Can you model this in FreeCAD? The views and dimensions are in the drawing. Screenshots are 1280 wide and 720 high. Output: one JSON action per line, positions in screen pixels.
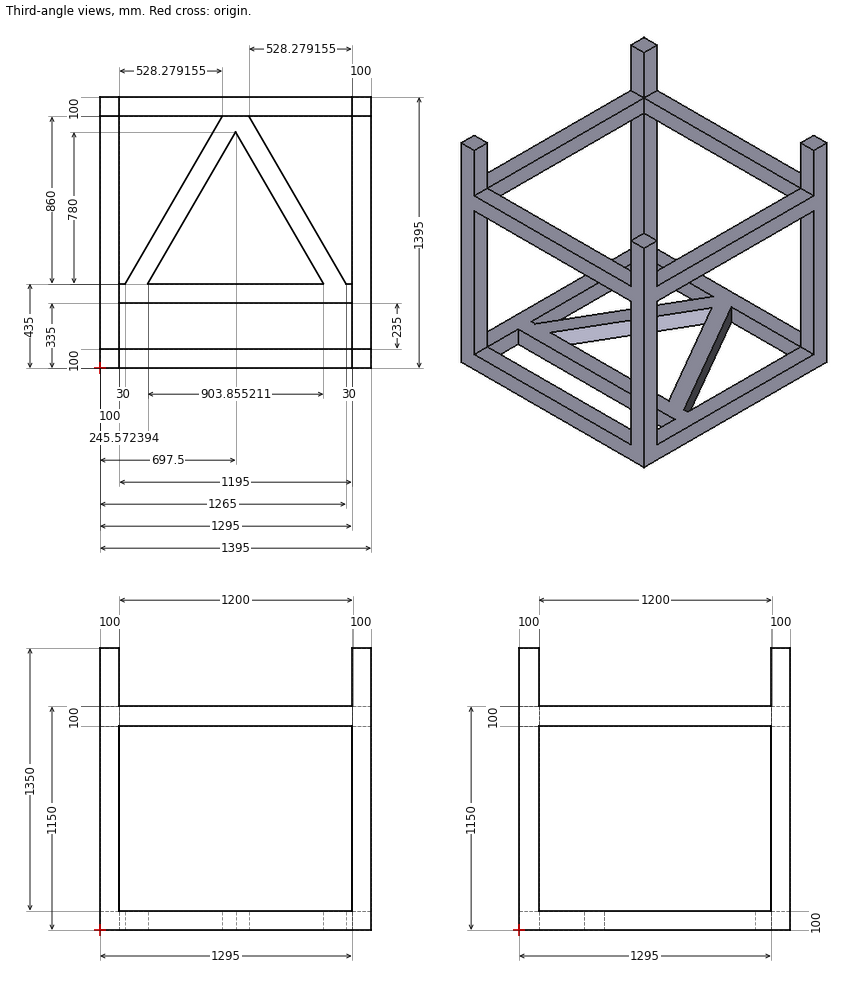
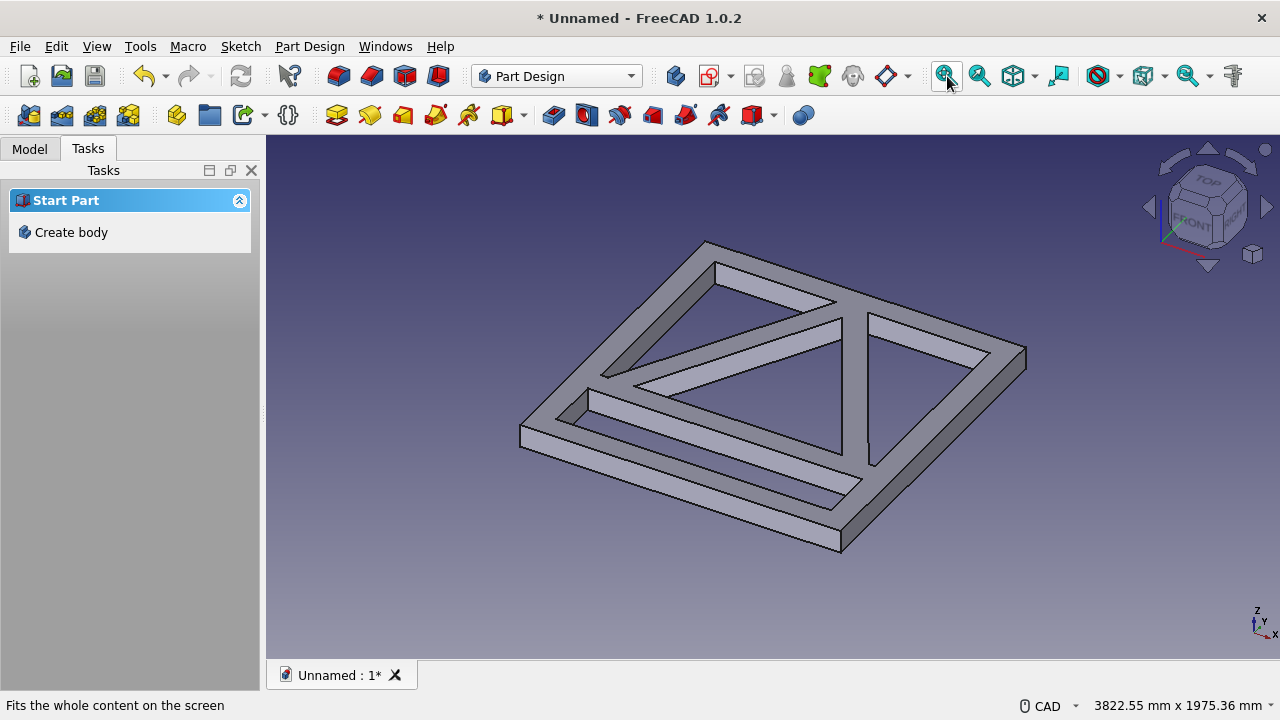
{"action": "left_click", "coordinate": [852, 306]}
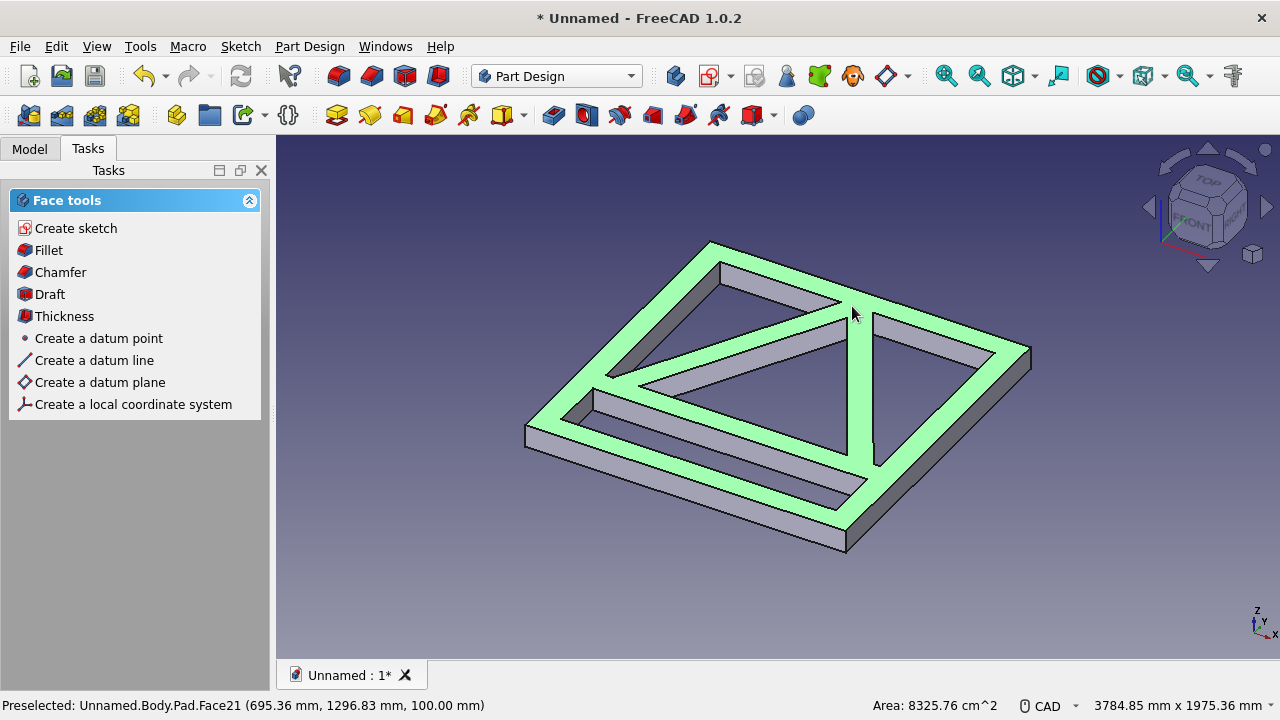
{"action": "left_click", "coordinate": [708, 76]}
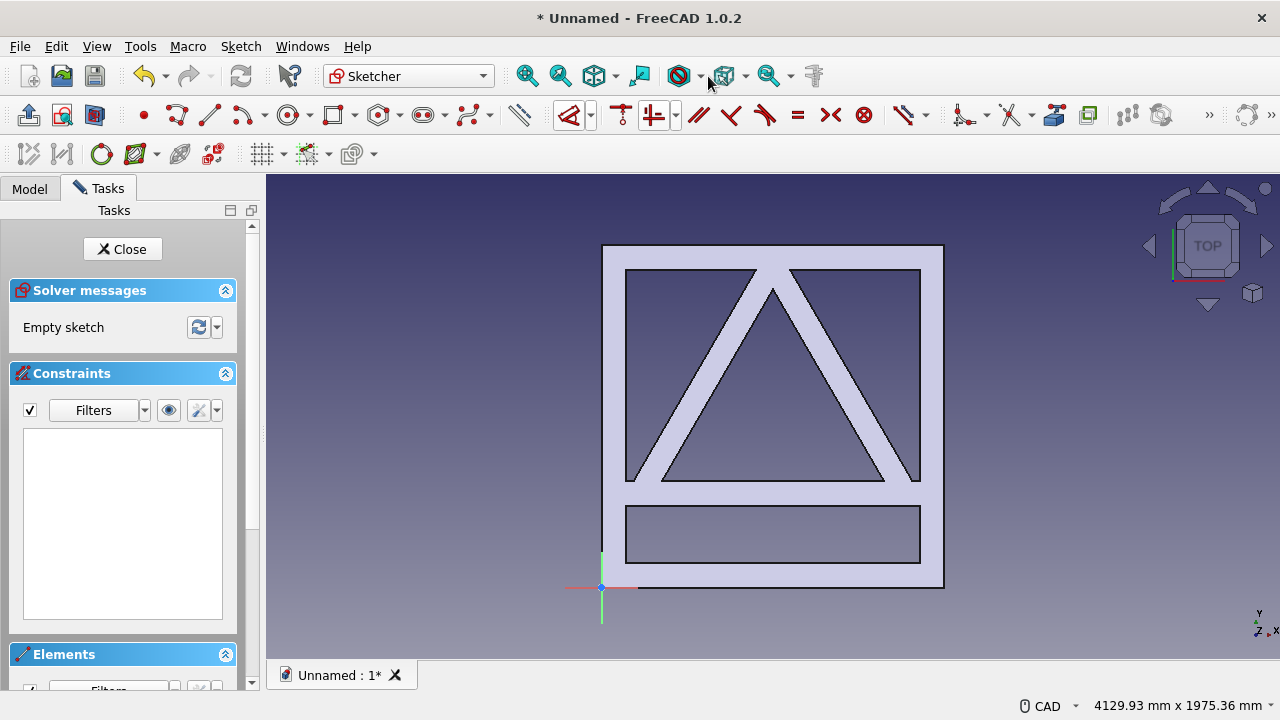
{"action": "left_click", "coordinate": [332, 116]}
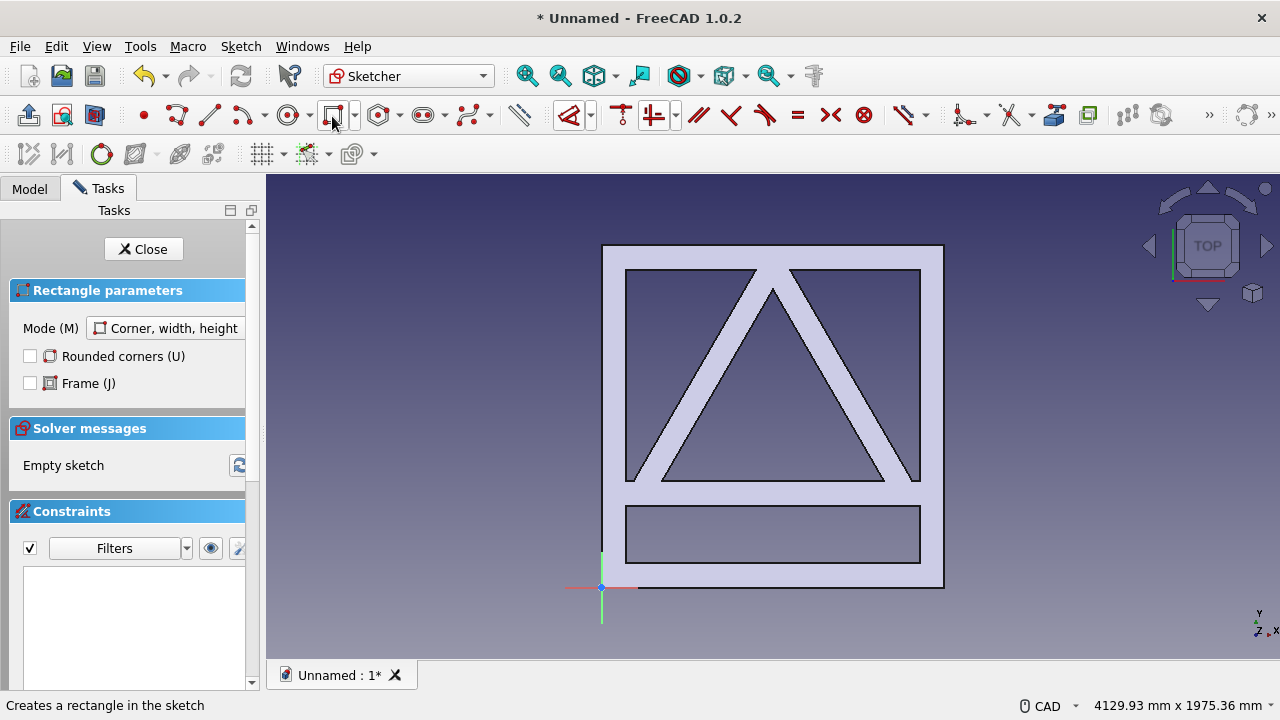
{"action": "left_click", "coordinate": [602, 245]}
{"action": "mouse_move", "coordinate": [626, 270]}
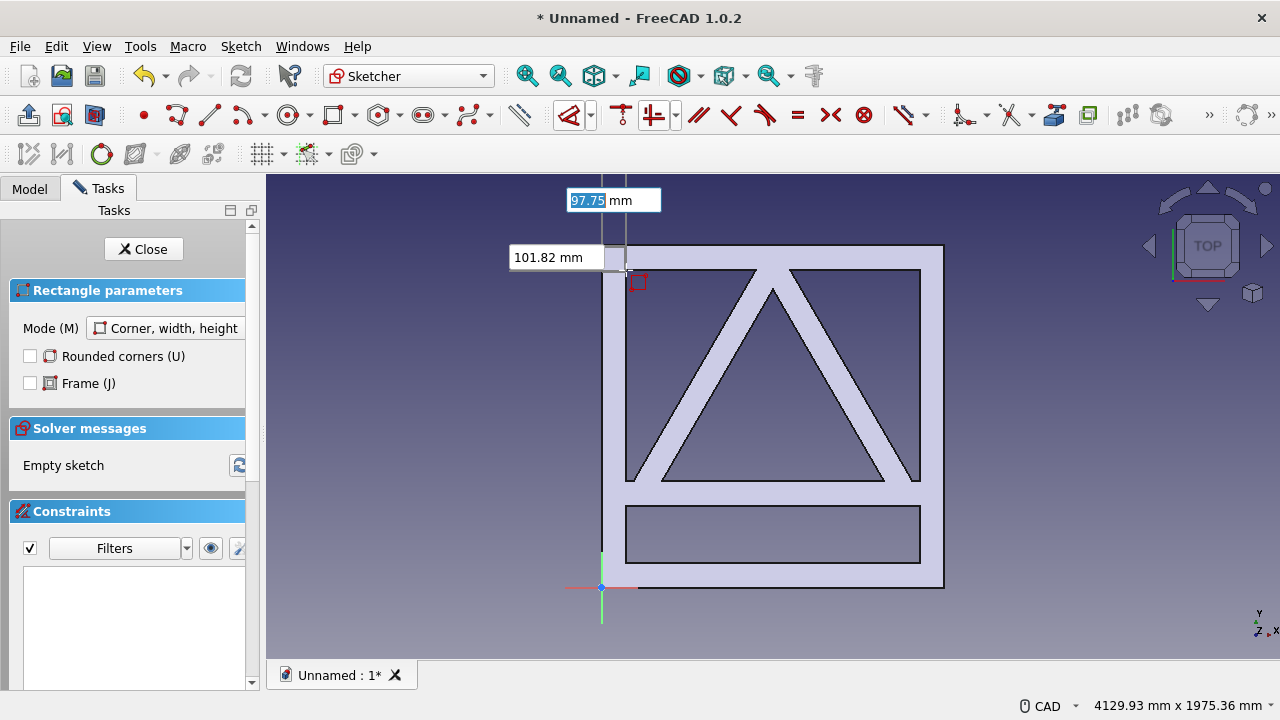
{"action": "type", "text": "100"}
{"action": "key", "text": "Tab"}
{"action": "type", "text": "100"}
{"action": "key", "text": "Return"}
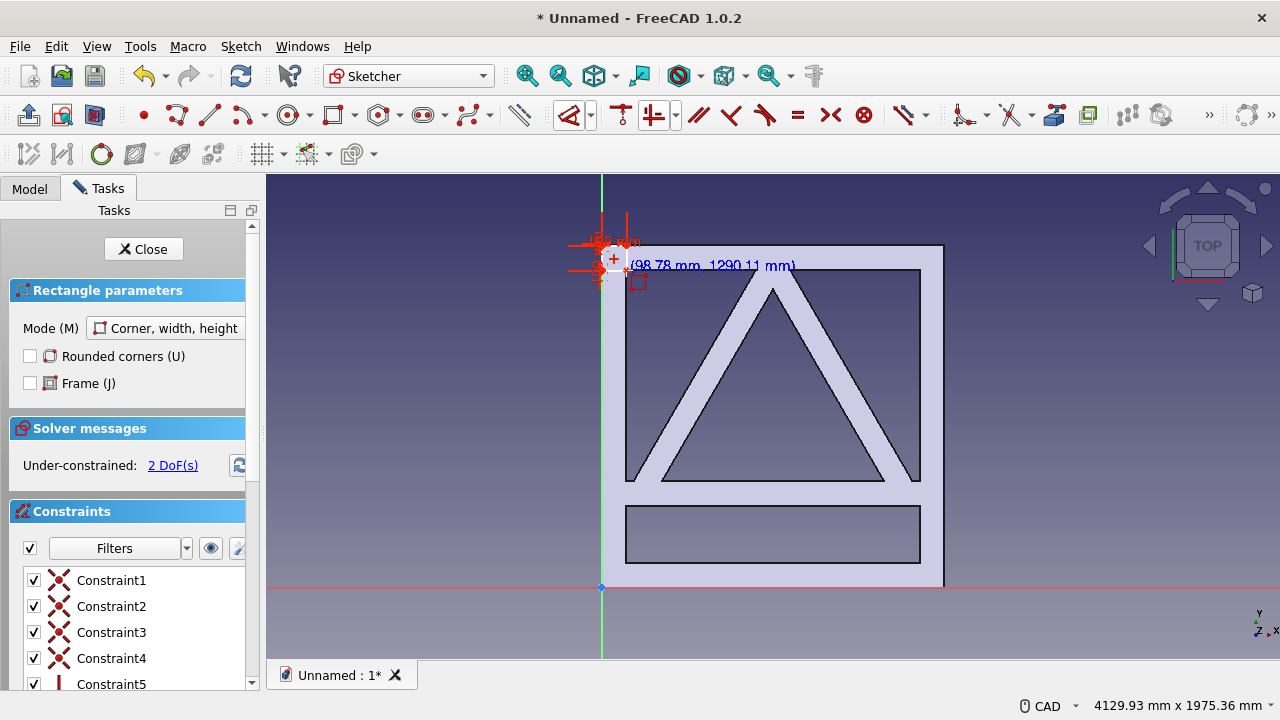
{"action": "left_click", "coordinate": [920, 245]}
{"action": "mouse_move", "coordinate": [944, 270]}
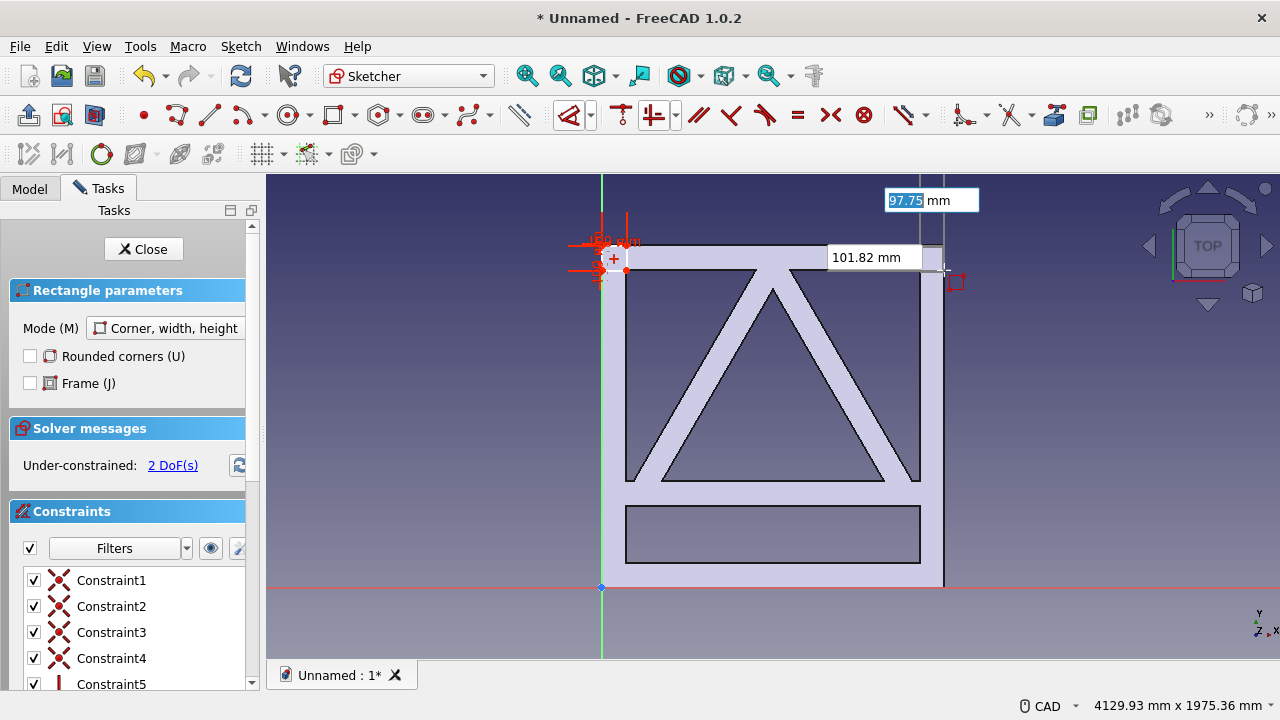
{"action": "type", "text": "100"}
{"action": "key", "text": "Tab"}
{"action": "type", "text": "100"}
{"action": "key", "text": "Return"}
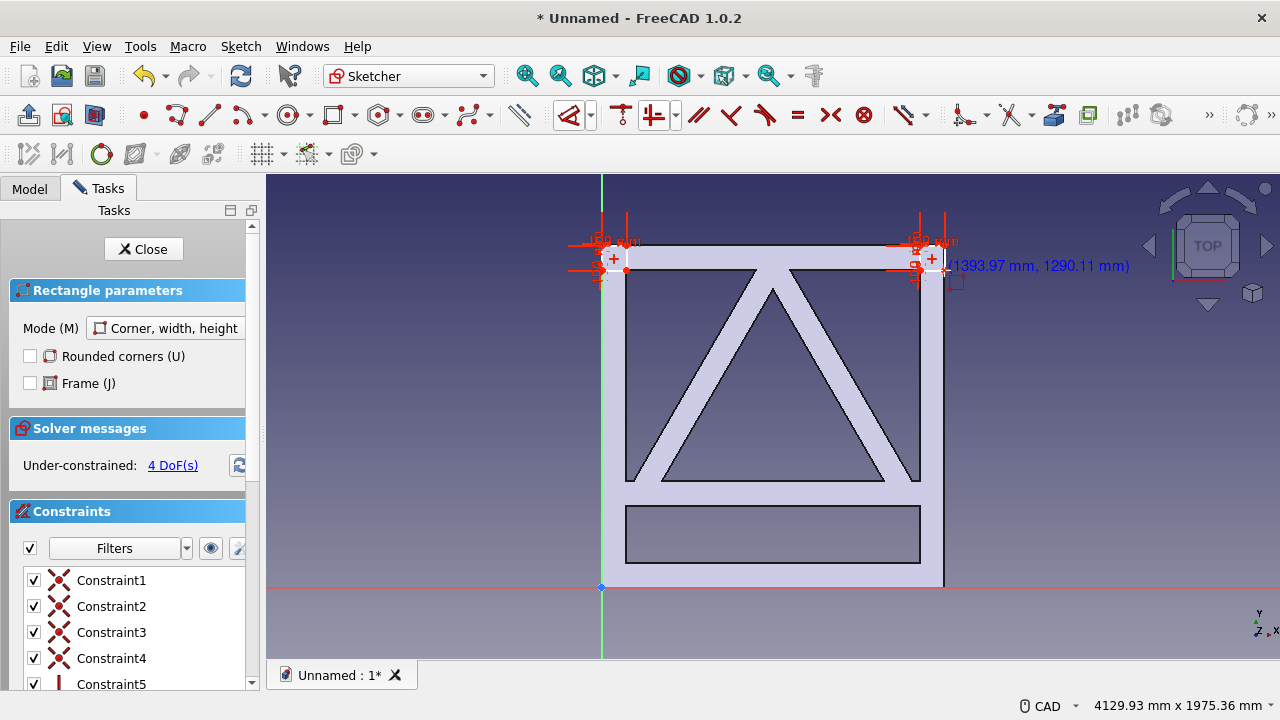
{"action": "left_click", "coordinate": [602, 588]}
{"action": "mouse_move", "coordinate": [626, 563]}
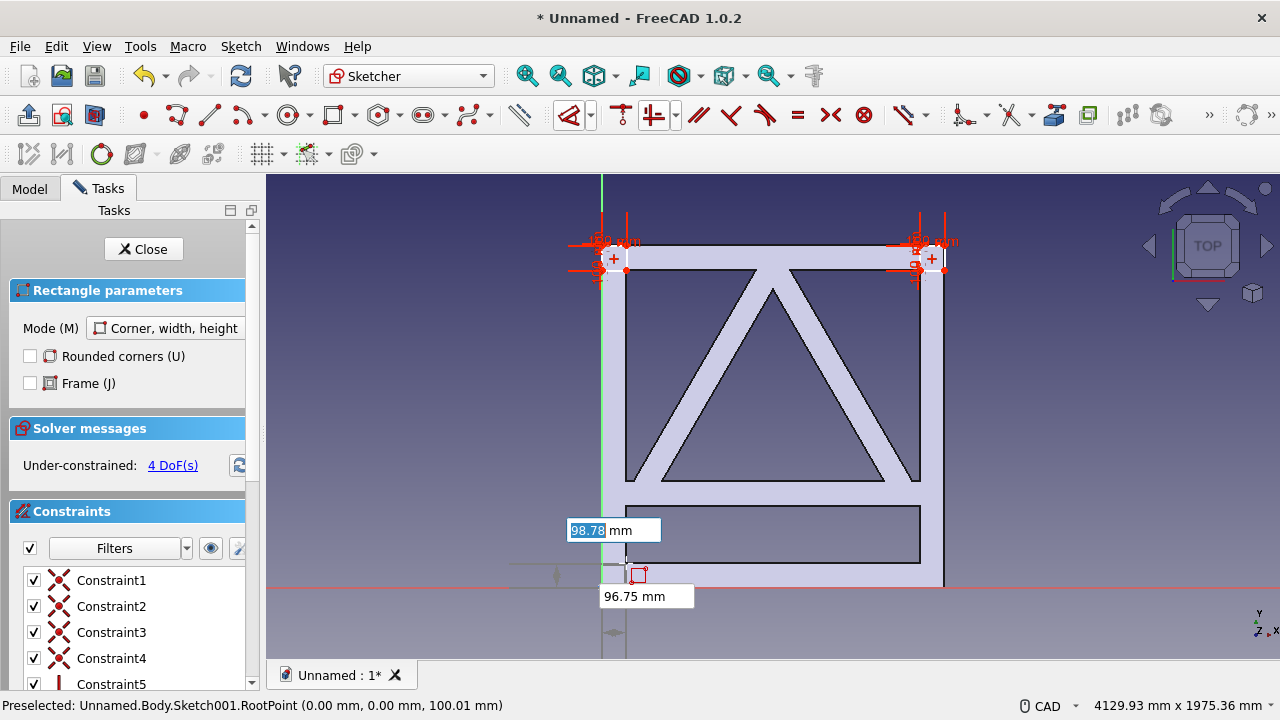
{"action": "type", "text": "100"}
{"action": "key", "text": "Tab"}
{"action": "type", "text": "100"}
{"action": "key", "text": "Return"}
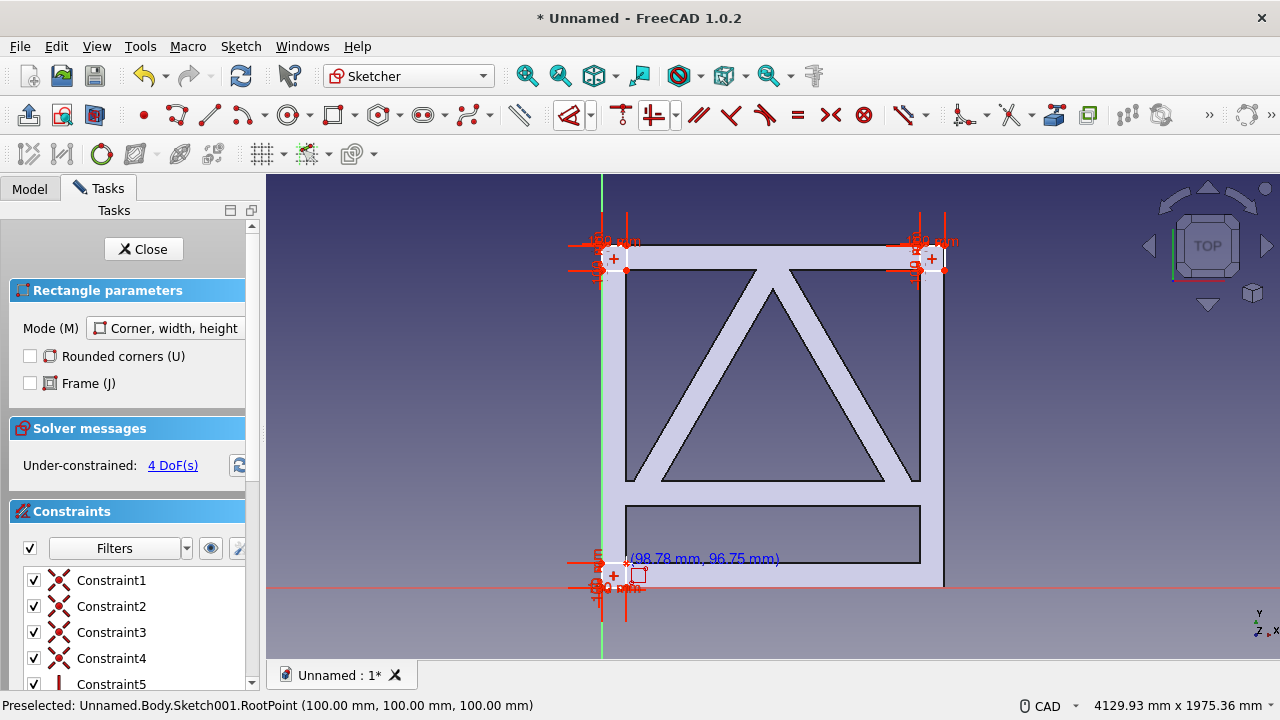
{"action": "left_click", "coordinate": [920, 563]}
{"action": "left_click", "coordinate": [944, 588]}
{"action": "key", "text": "Escape"}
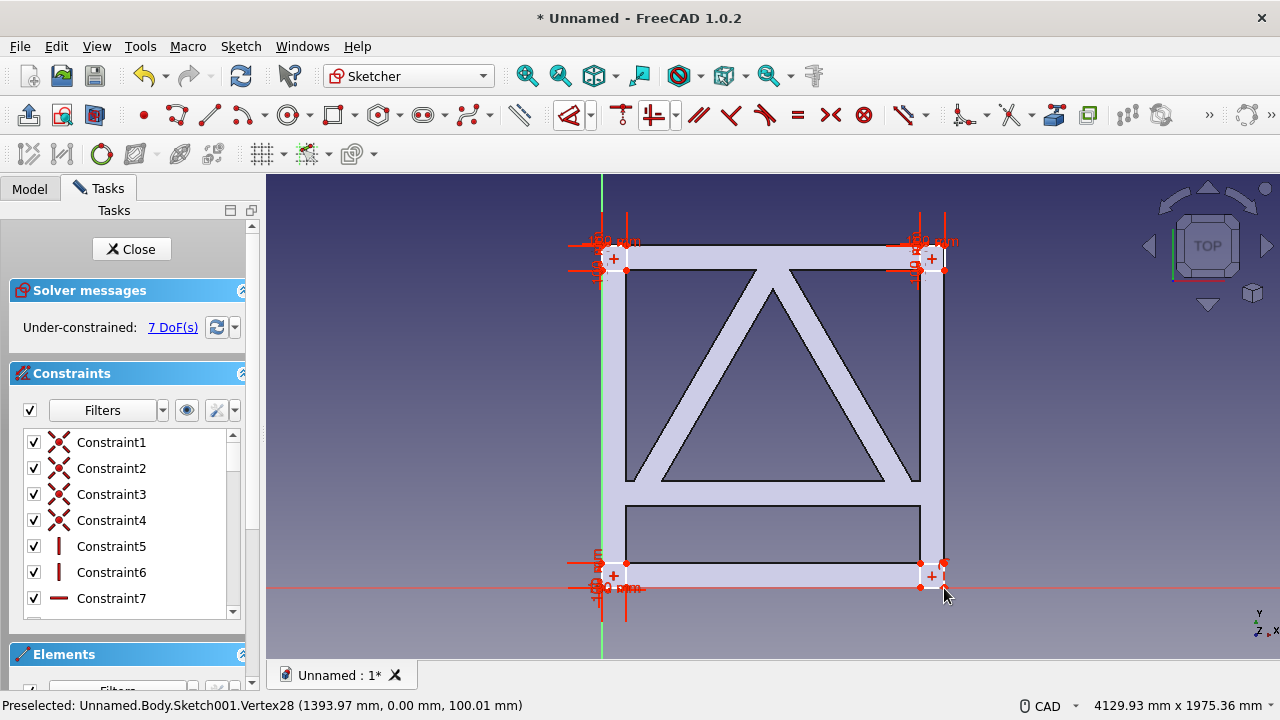
{"action": "left_click", "coordinate": [602, 246]}